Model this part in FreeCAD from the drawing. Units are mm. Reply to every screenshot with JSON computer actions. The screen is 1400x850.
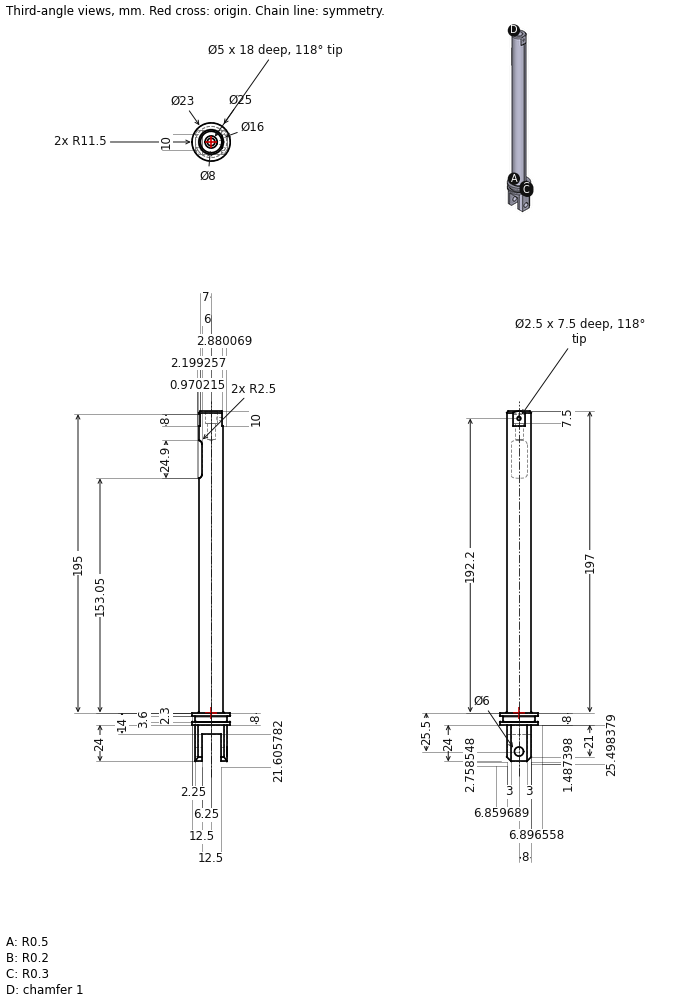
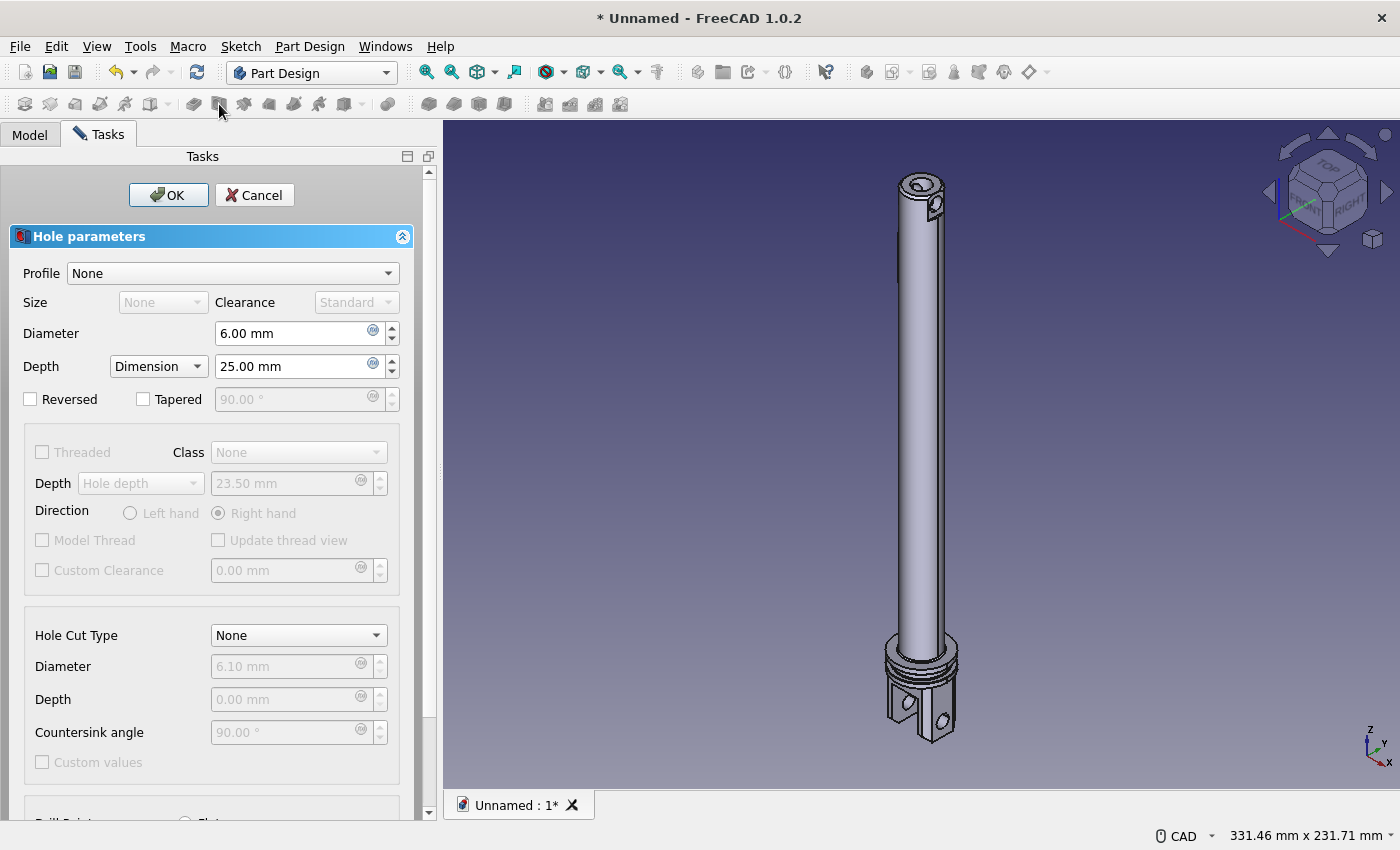
{"action": "triple_click", "coordinate": [300, 334]}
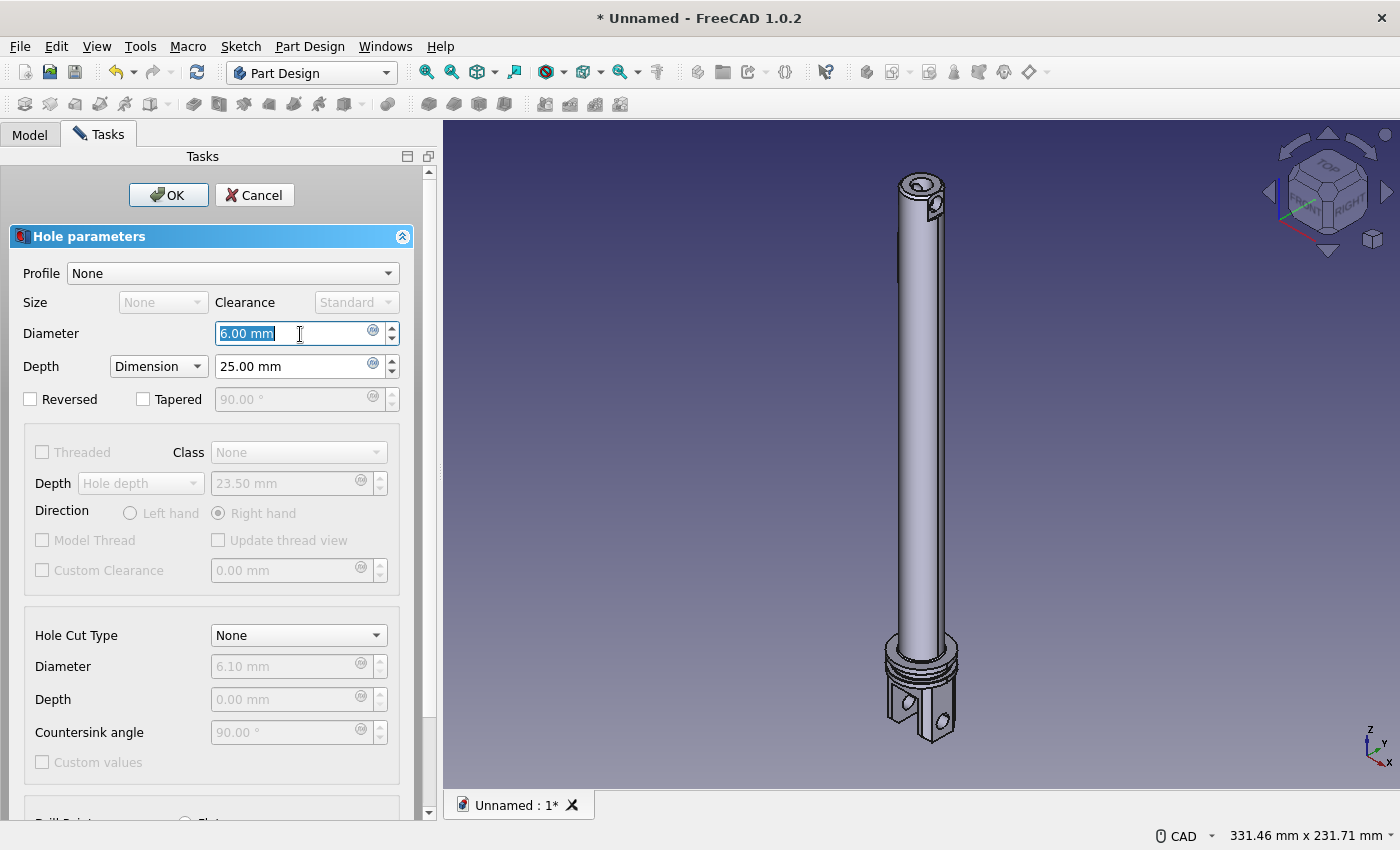
{"action": "type", "text": "2.5"}
{"action": "key", "text": "Tab"}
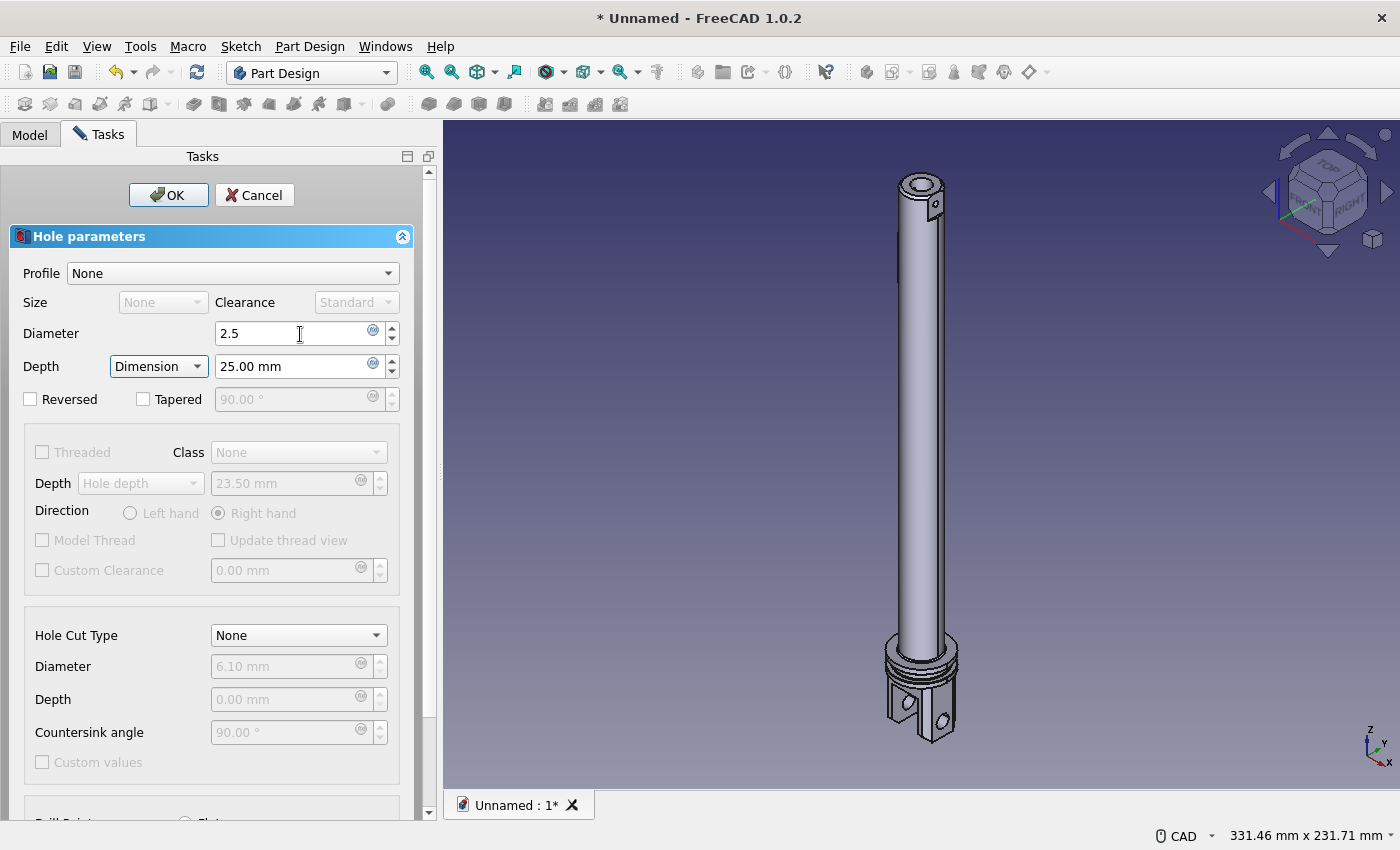
{"action": "triple_click", "coordinate": [300, 366]}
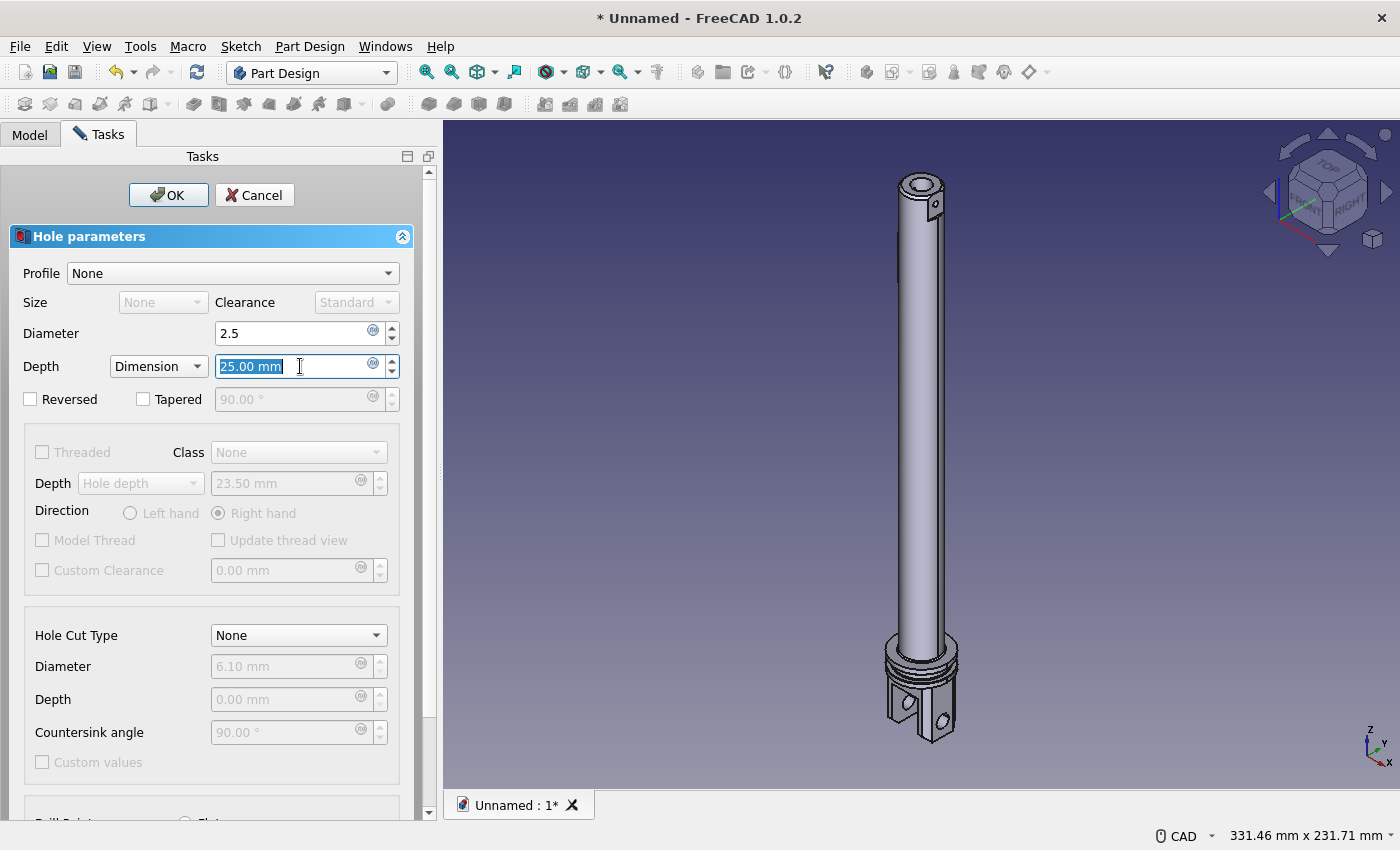
{"action": "type", "text": "7.5"}
{"action": "key", "text": "Tab"}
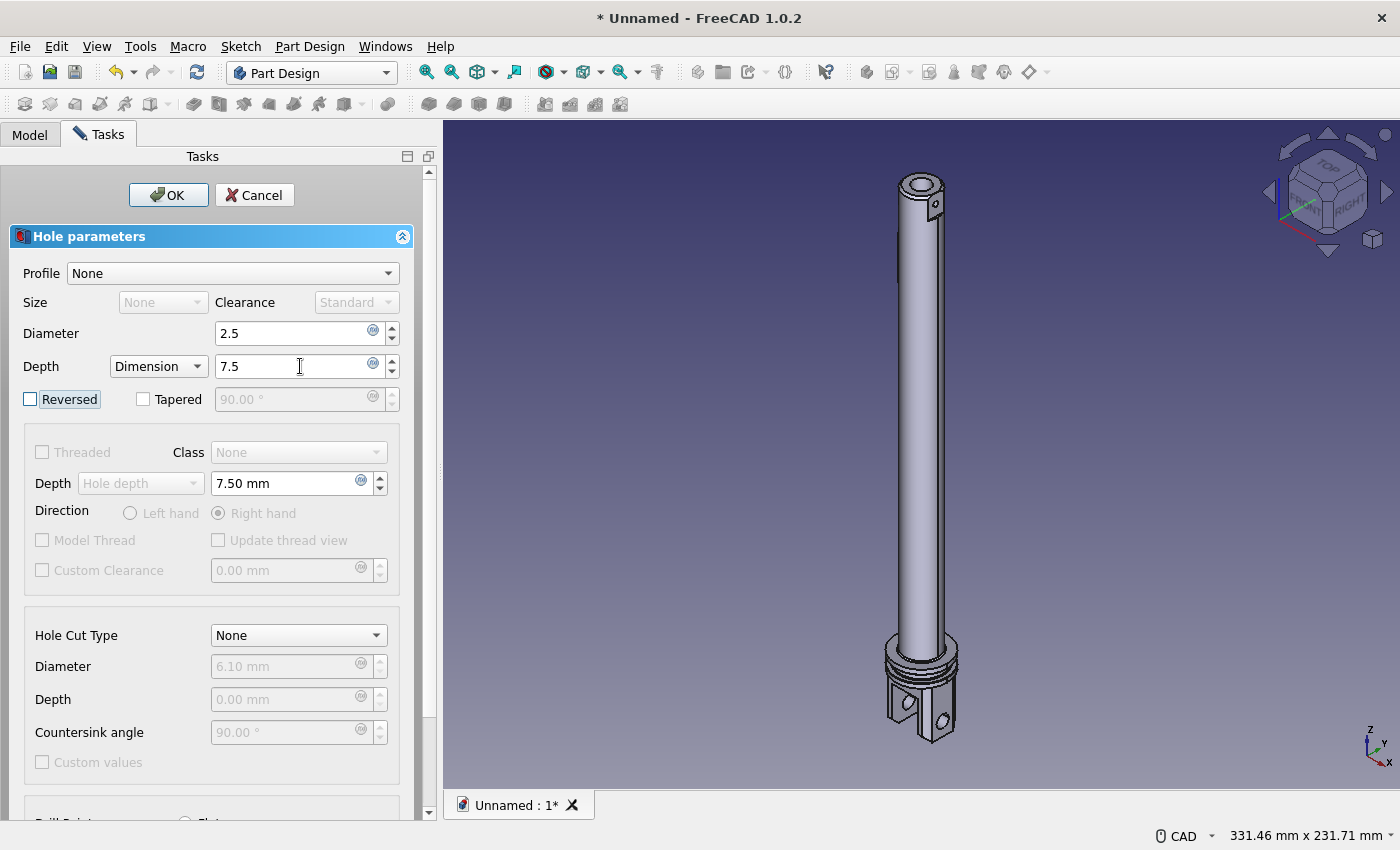
{"action": "left_click", "coordinate": [169, 195]}